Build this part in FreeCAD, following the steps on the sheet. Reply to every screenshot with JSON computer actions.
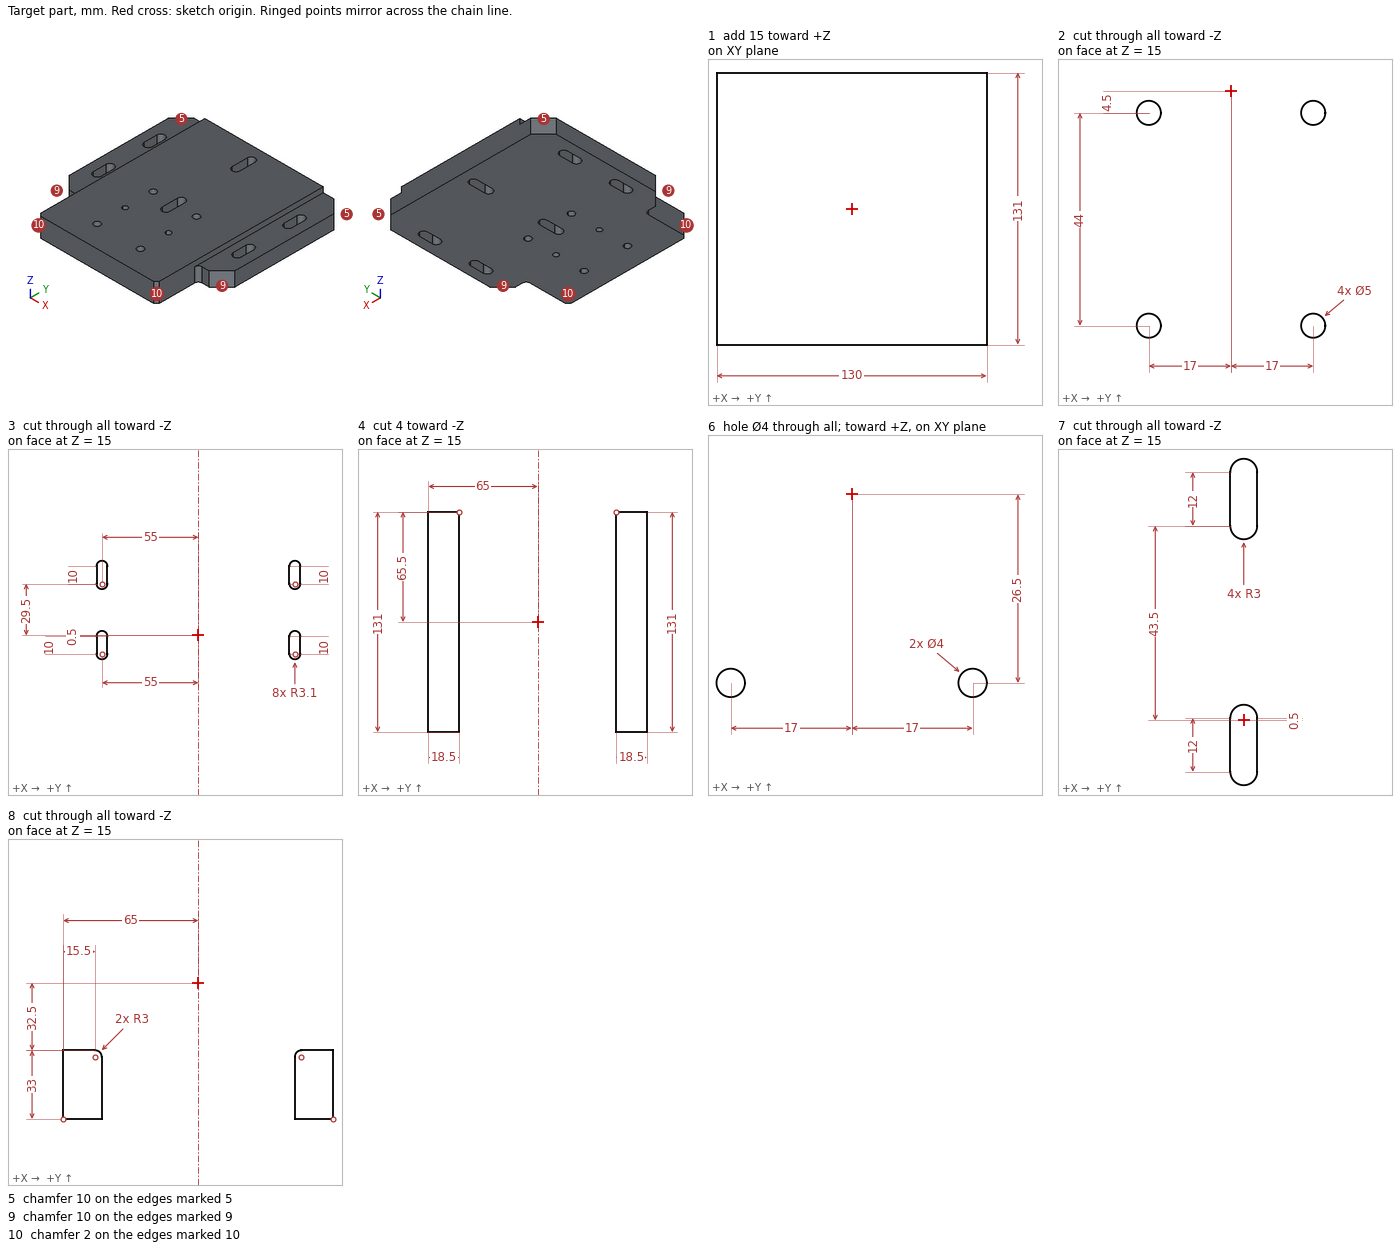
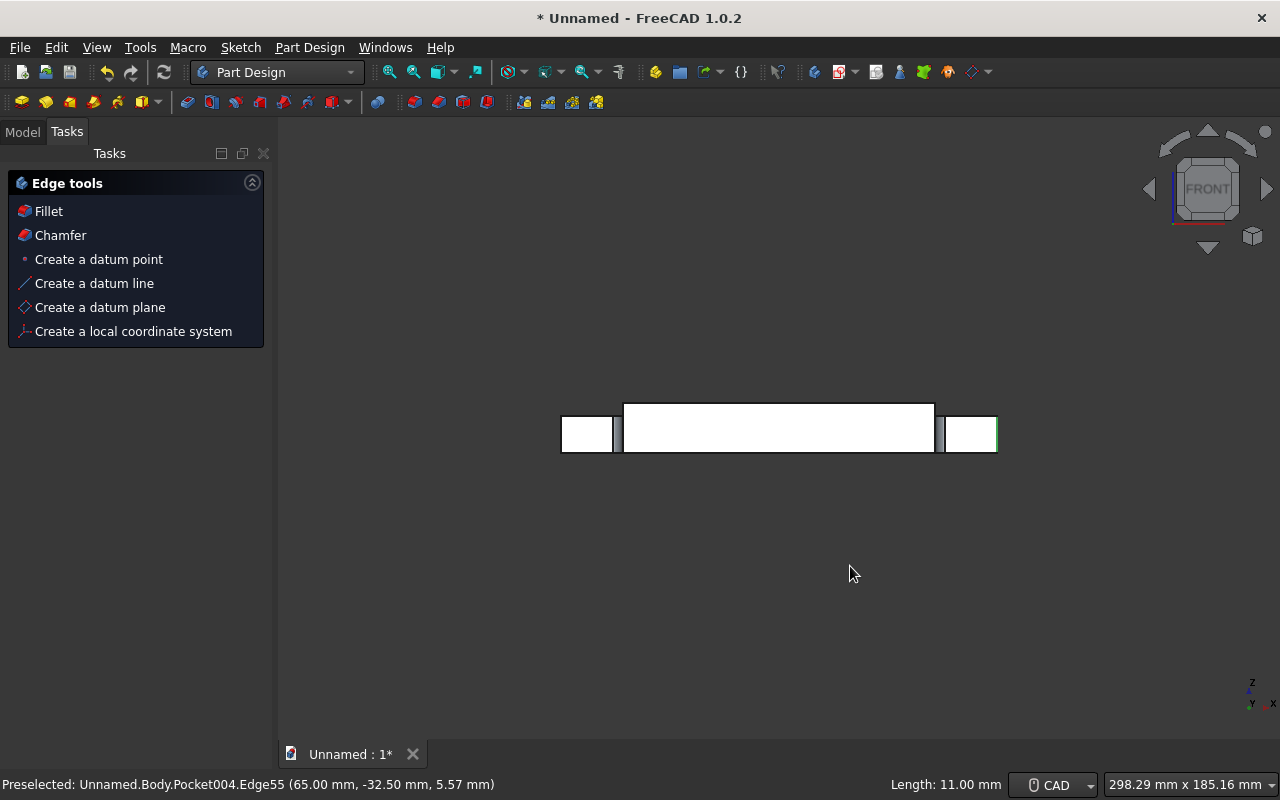
{"action": "left_click", "coordinate": [390, 72]}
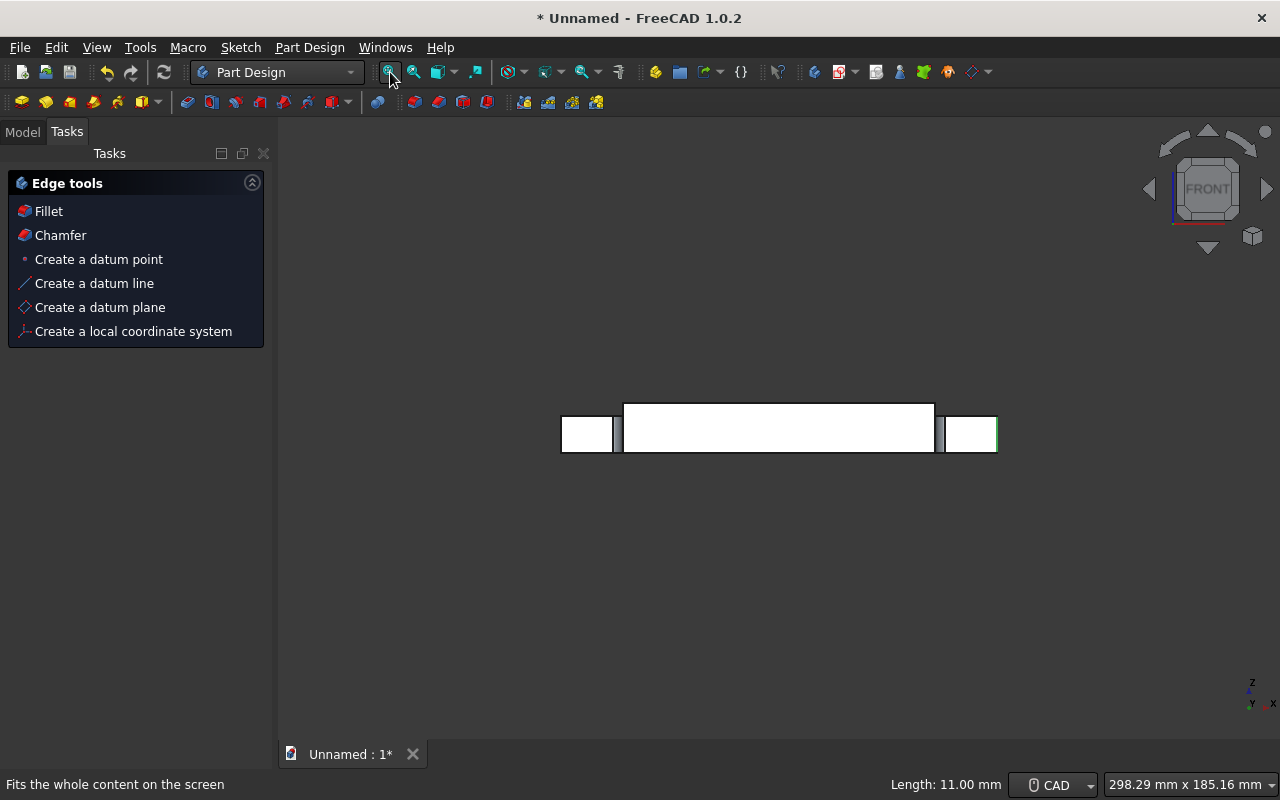
{"action": "left_click", "coordinate": [561, 434], "text": "ctrl"}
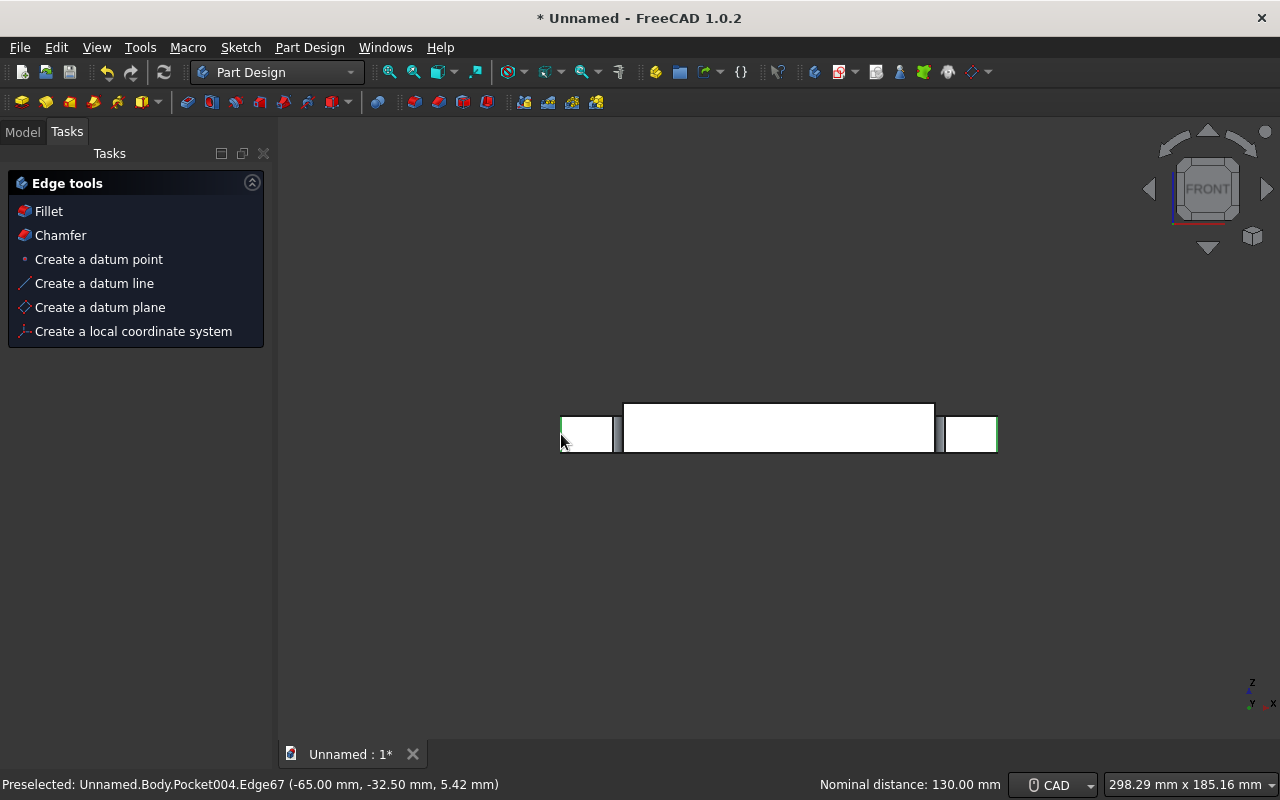
{"action": "left_click", "coordinate": [440, 102]}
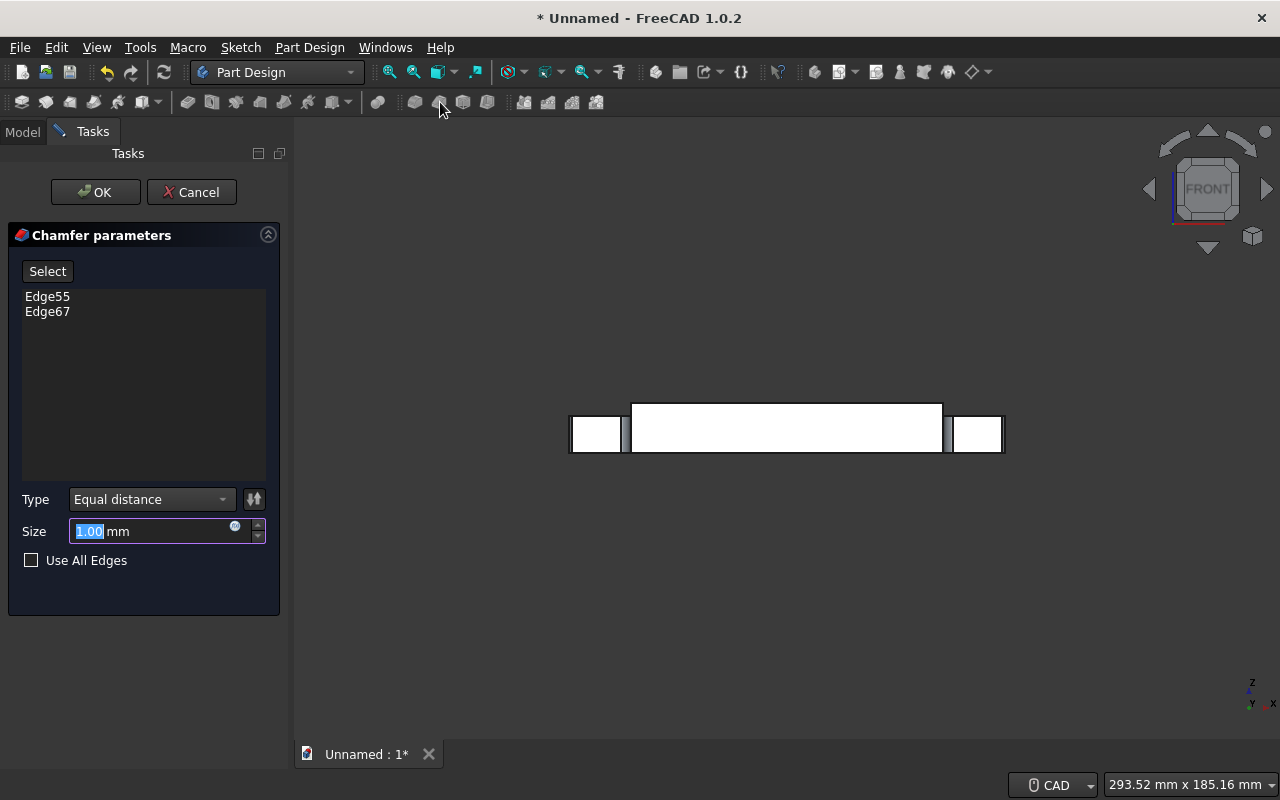
{"action": "type", "text": "10"}
{"action": "key", "text": "Tab"}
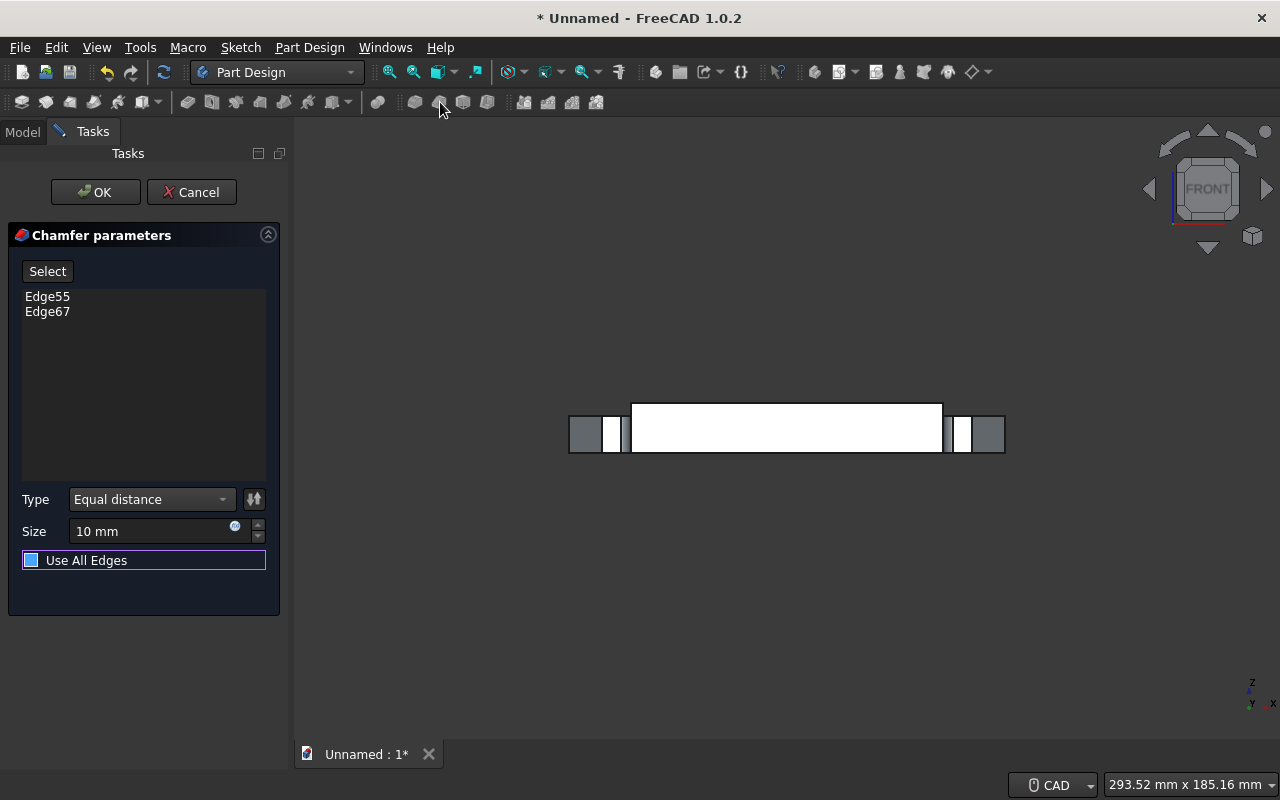
{"action": "left_click", "coordinate": [96, 192]}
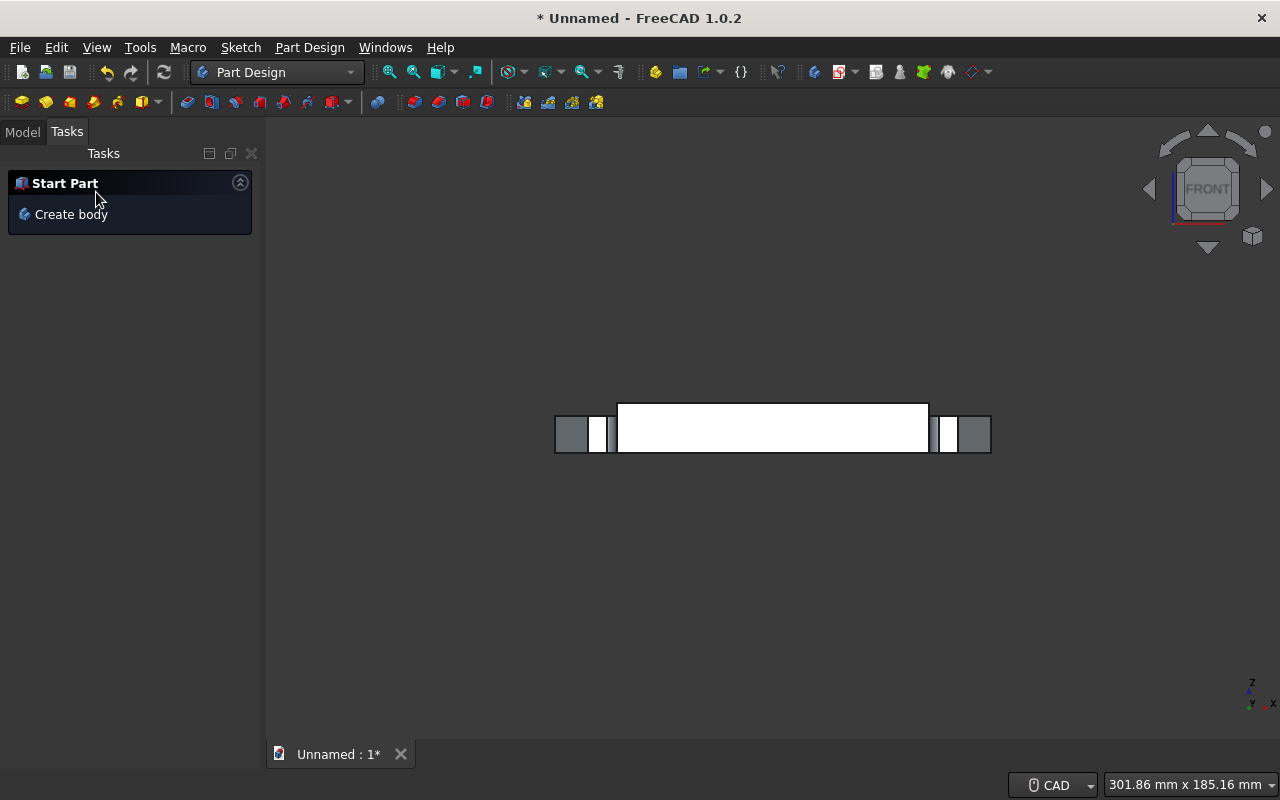
{"action": "key", "text": "v f"}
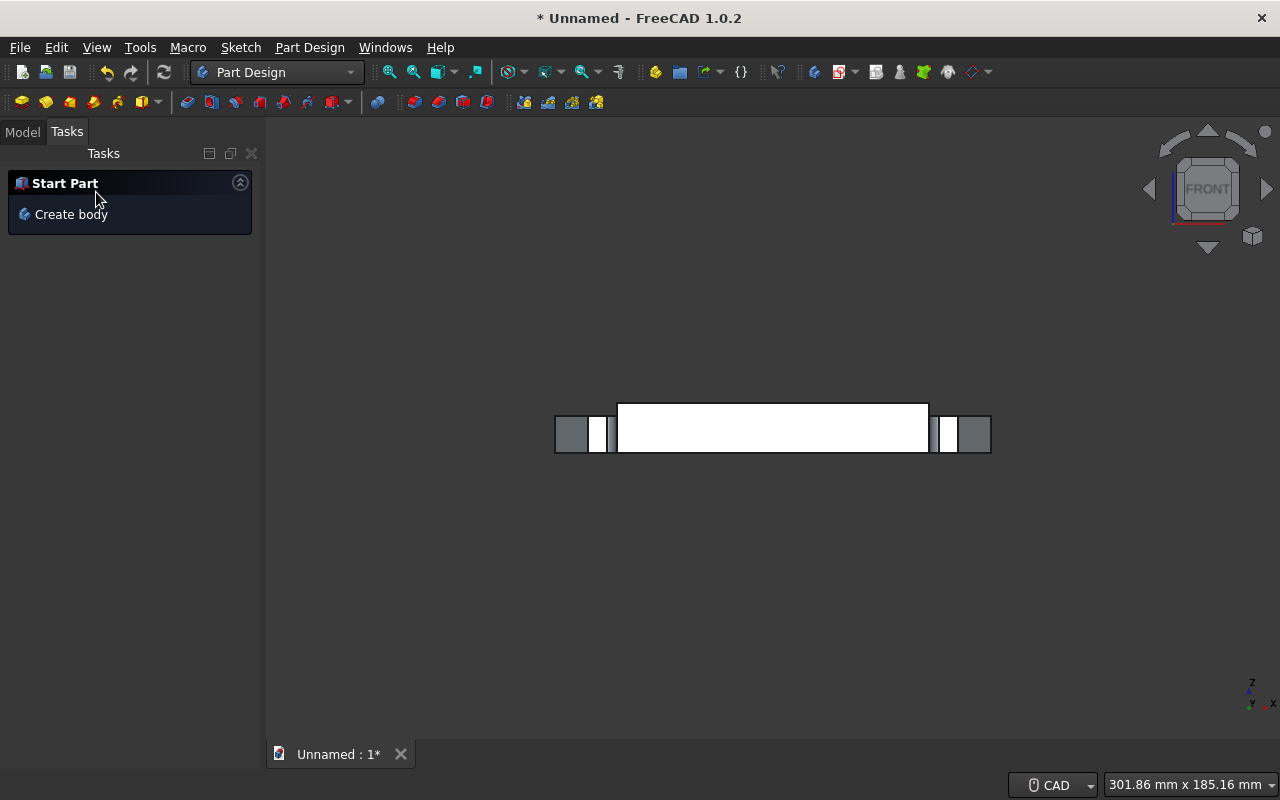
{"action": "left_click", "coordinate": [617, 427]}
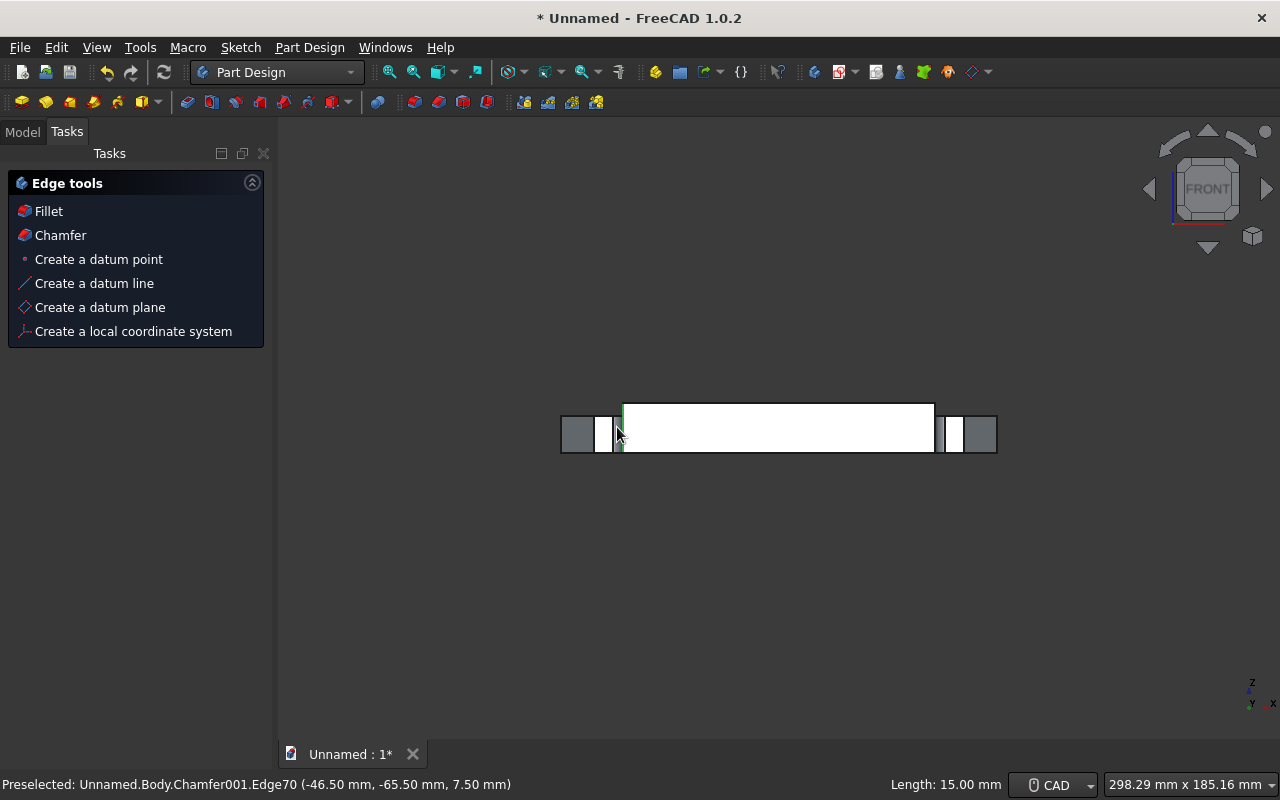
{"action": "left_click", "coordinate": [935, 427], "text": "ctrl"}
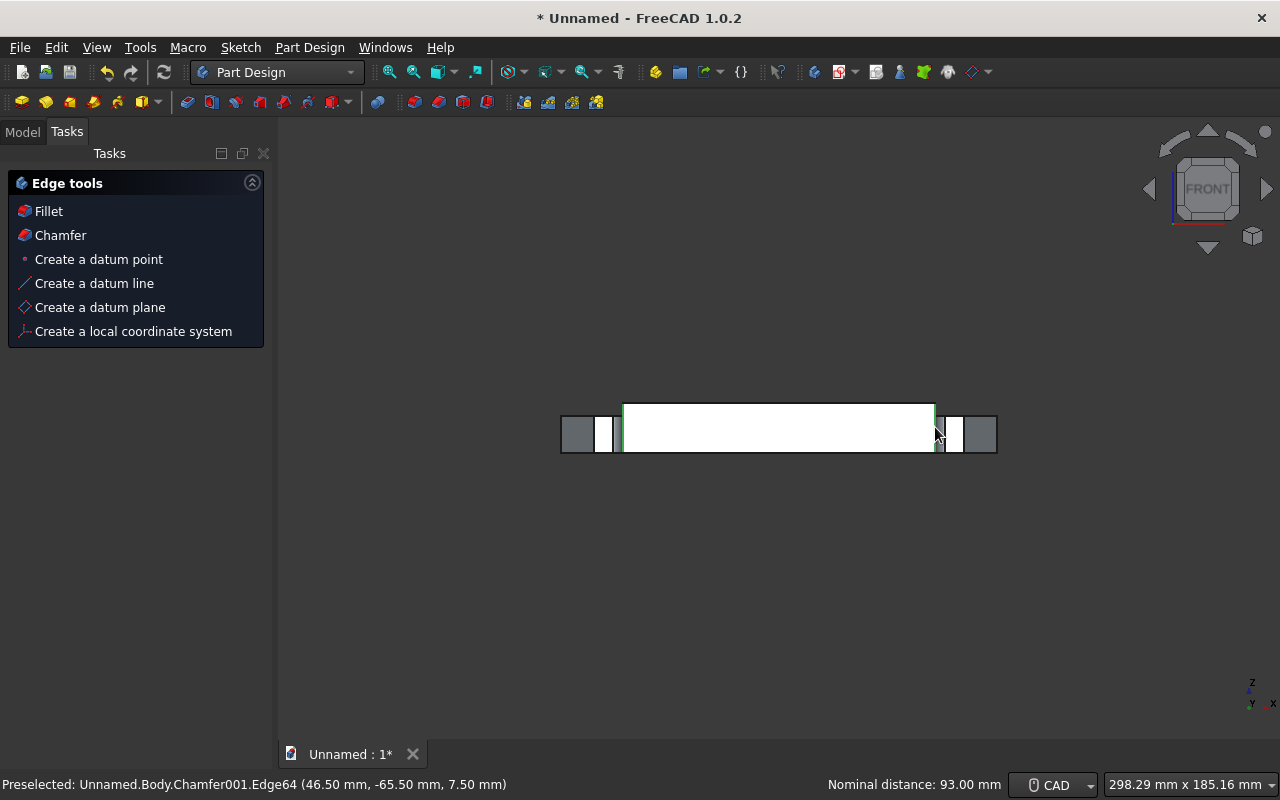
{"action": "left_click", "coordinate": [440, 102]}